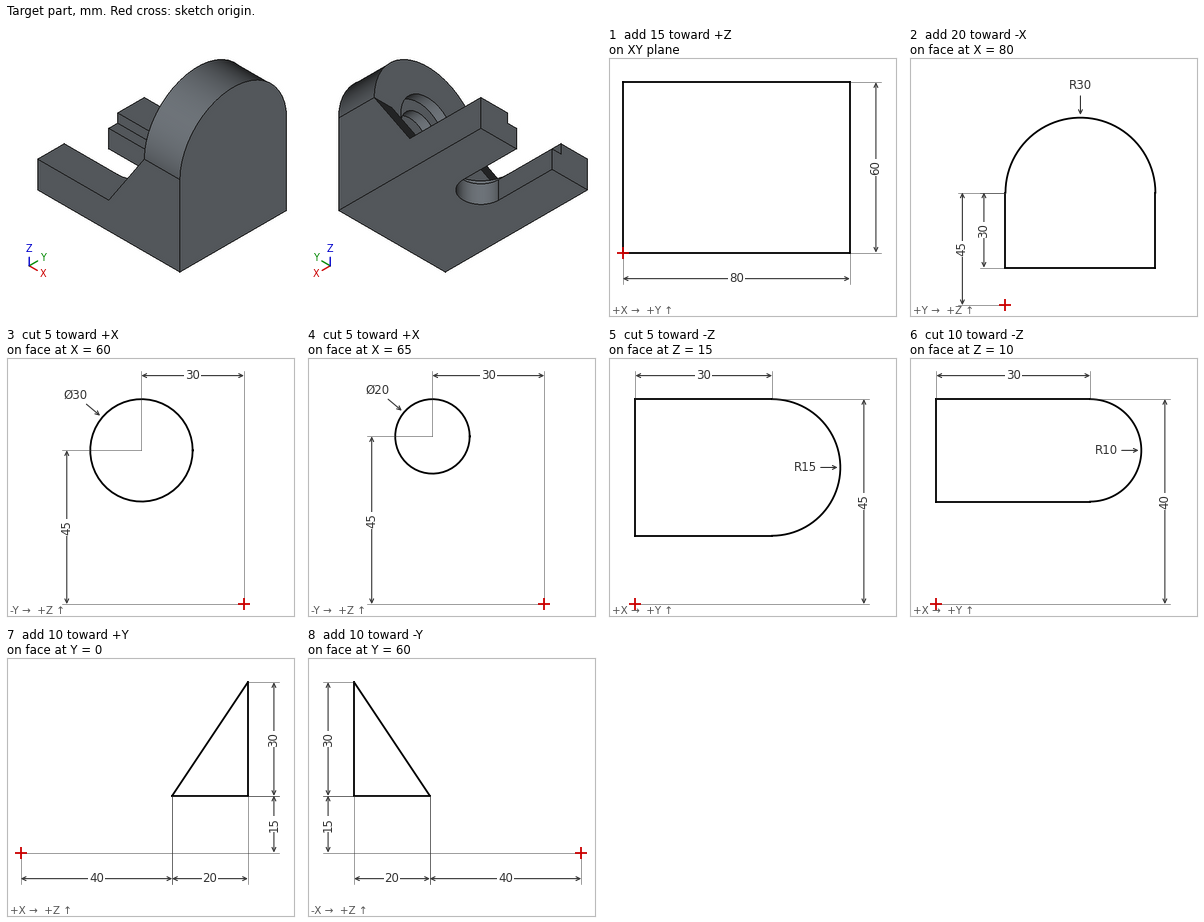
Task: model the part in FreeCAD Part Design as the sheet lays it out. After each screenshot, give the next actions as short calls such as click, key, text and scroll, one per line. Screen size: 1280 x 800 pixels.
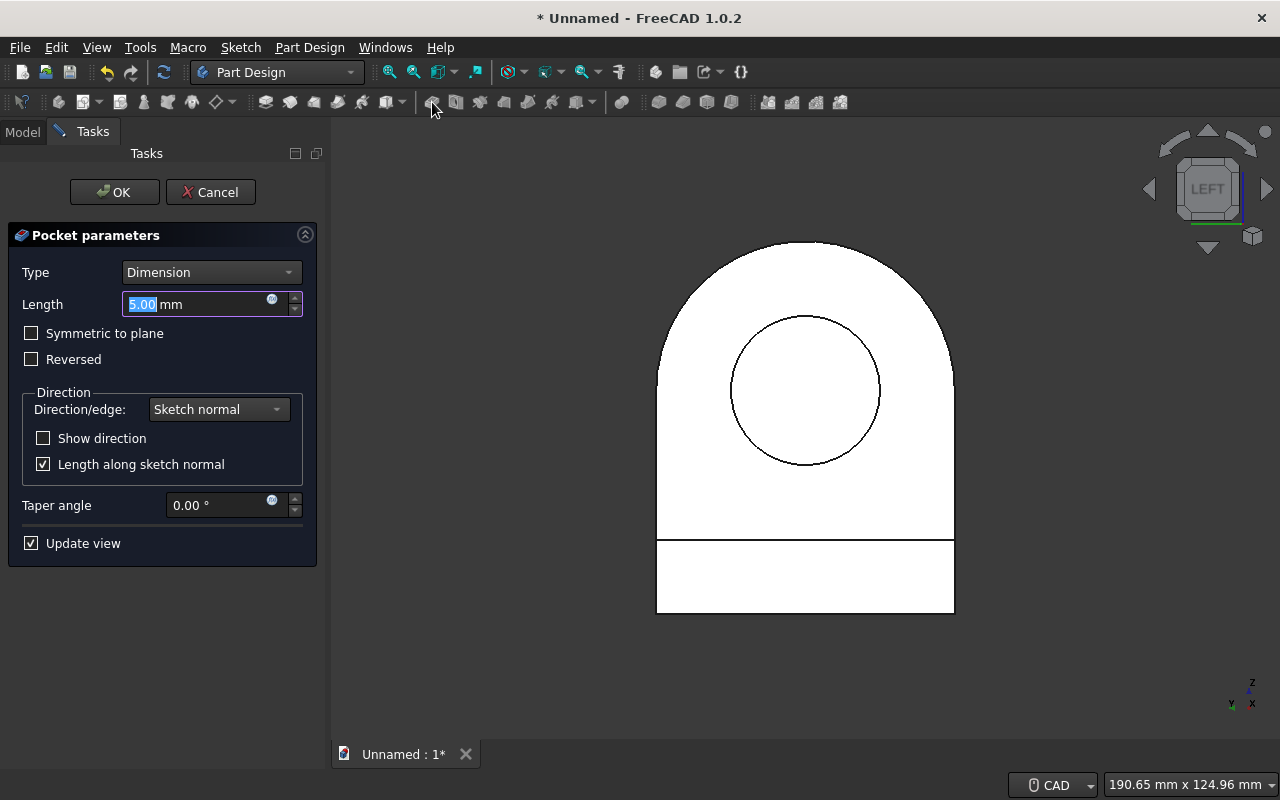
text(5)
key(Tab)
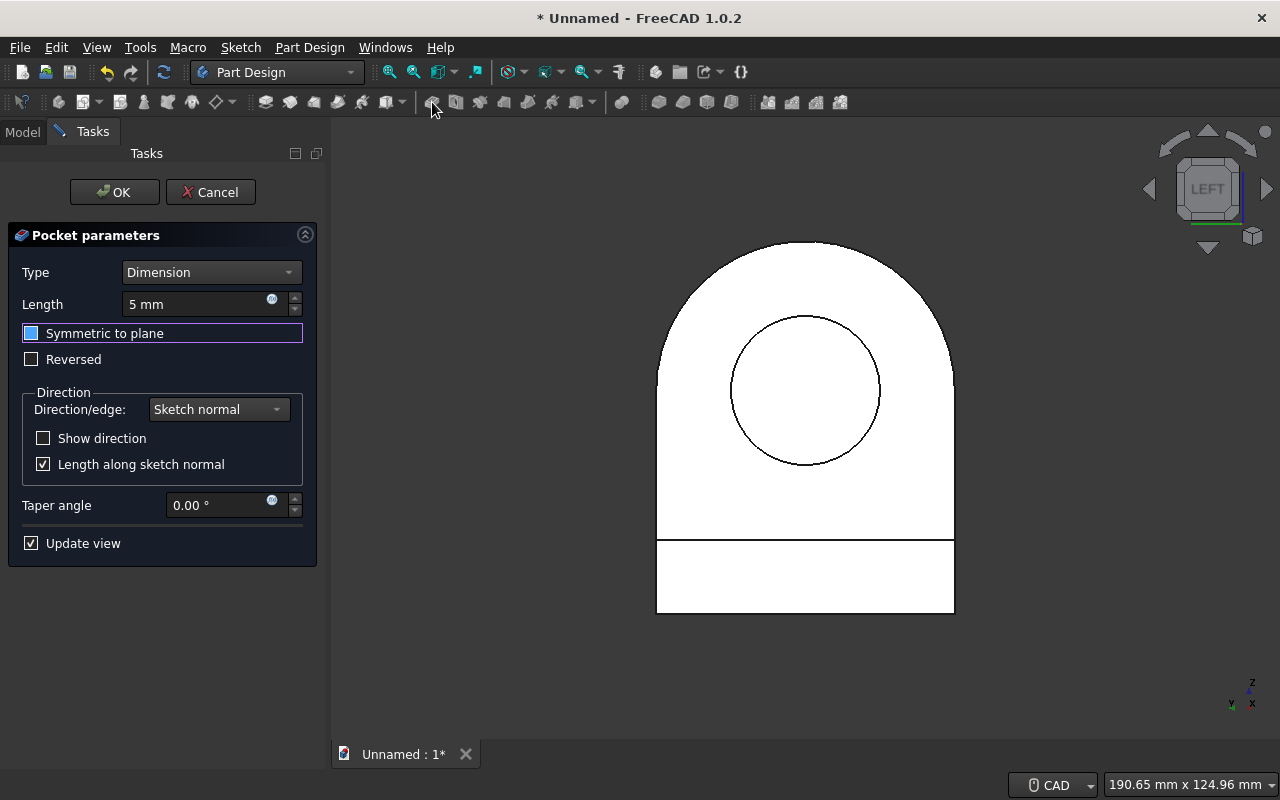
click(115, 192)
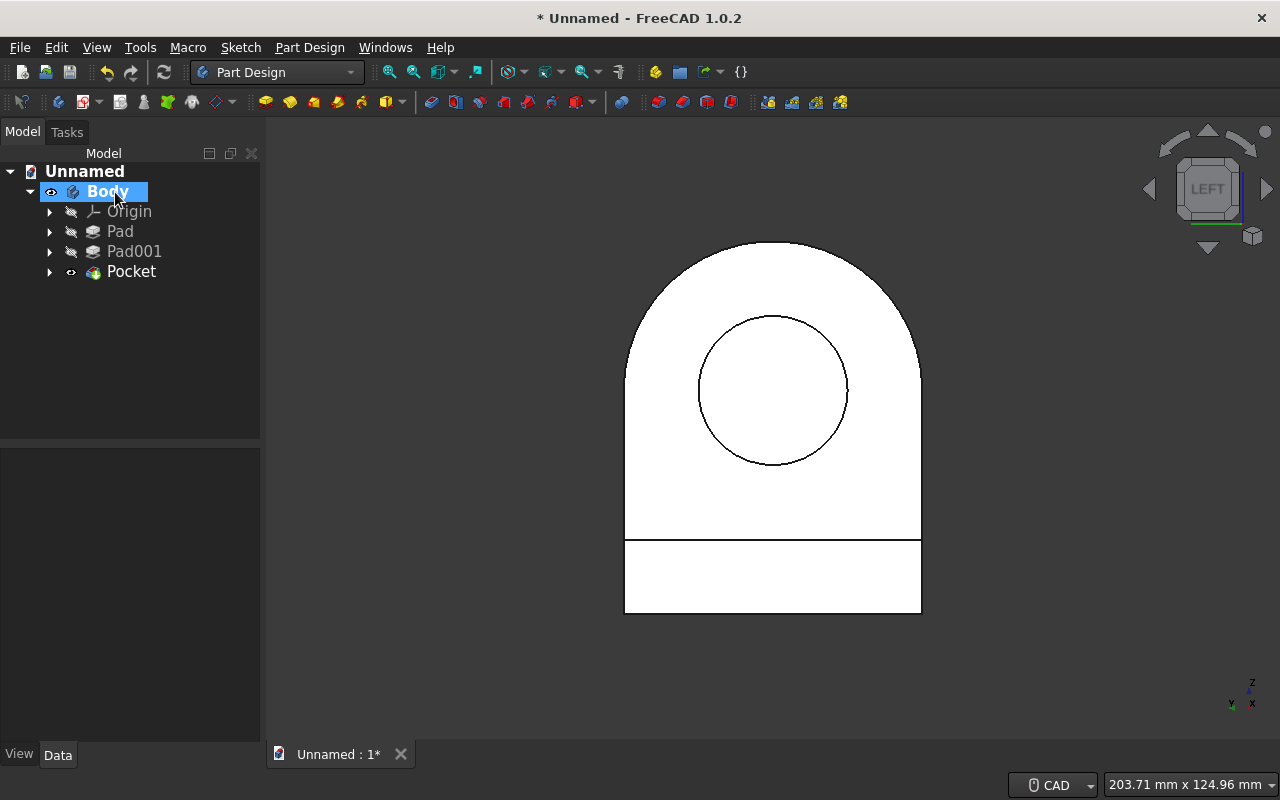
click(773, 389)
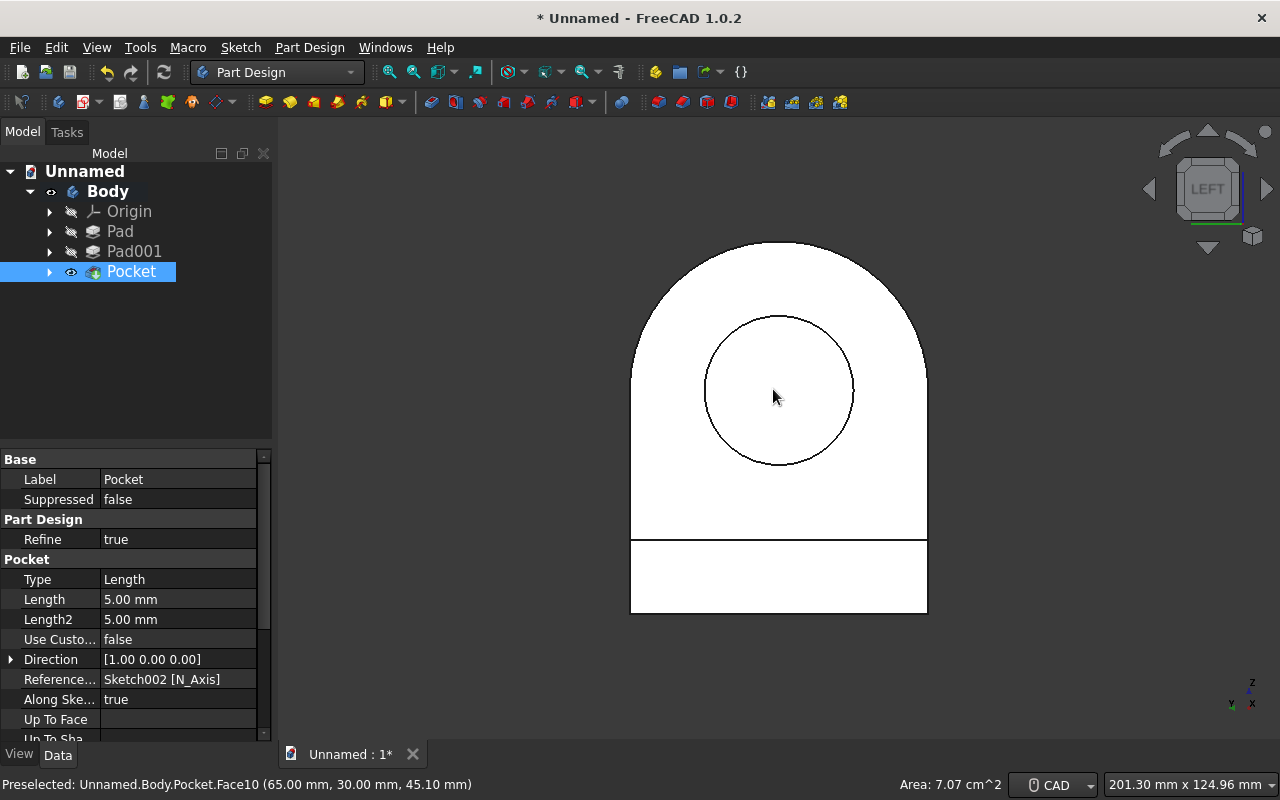
click(84, 102)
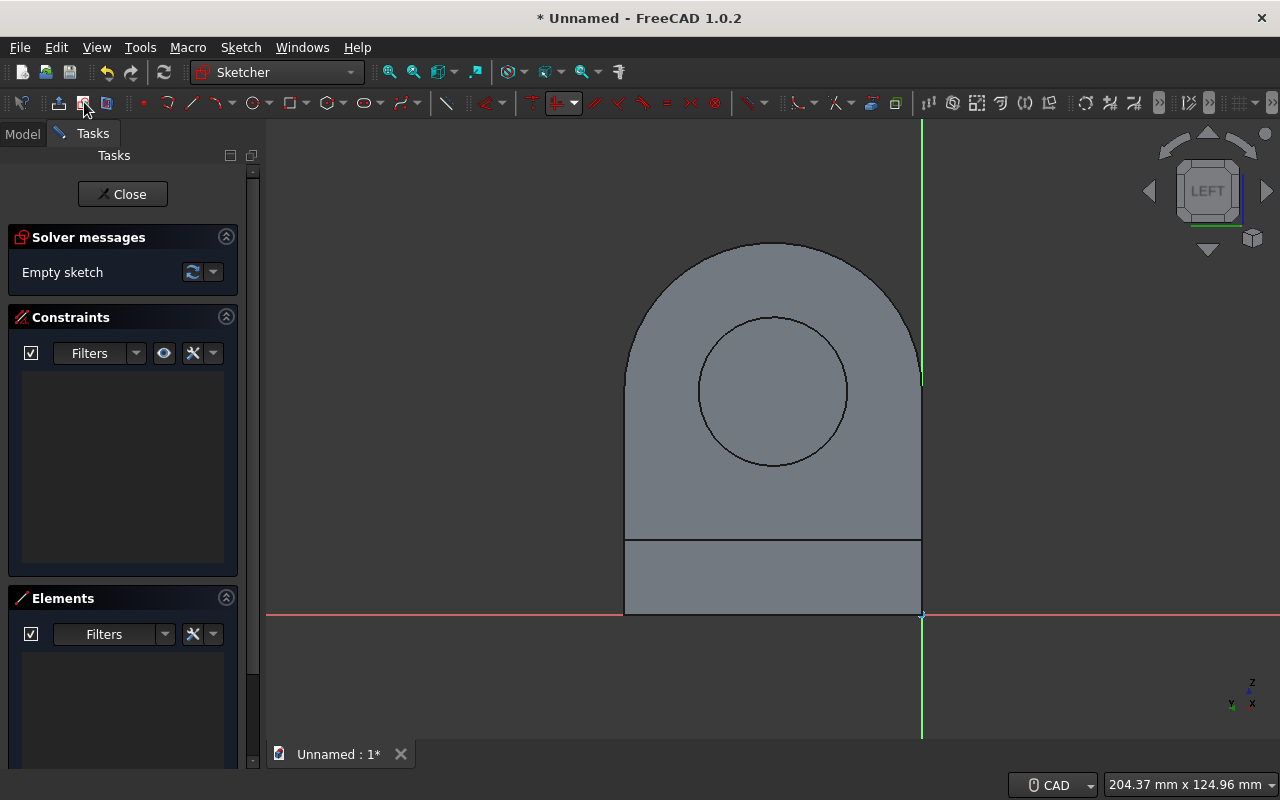
scroll(795, 379, up, 7)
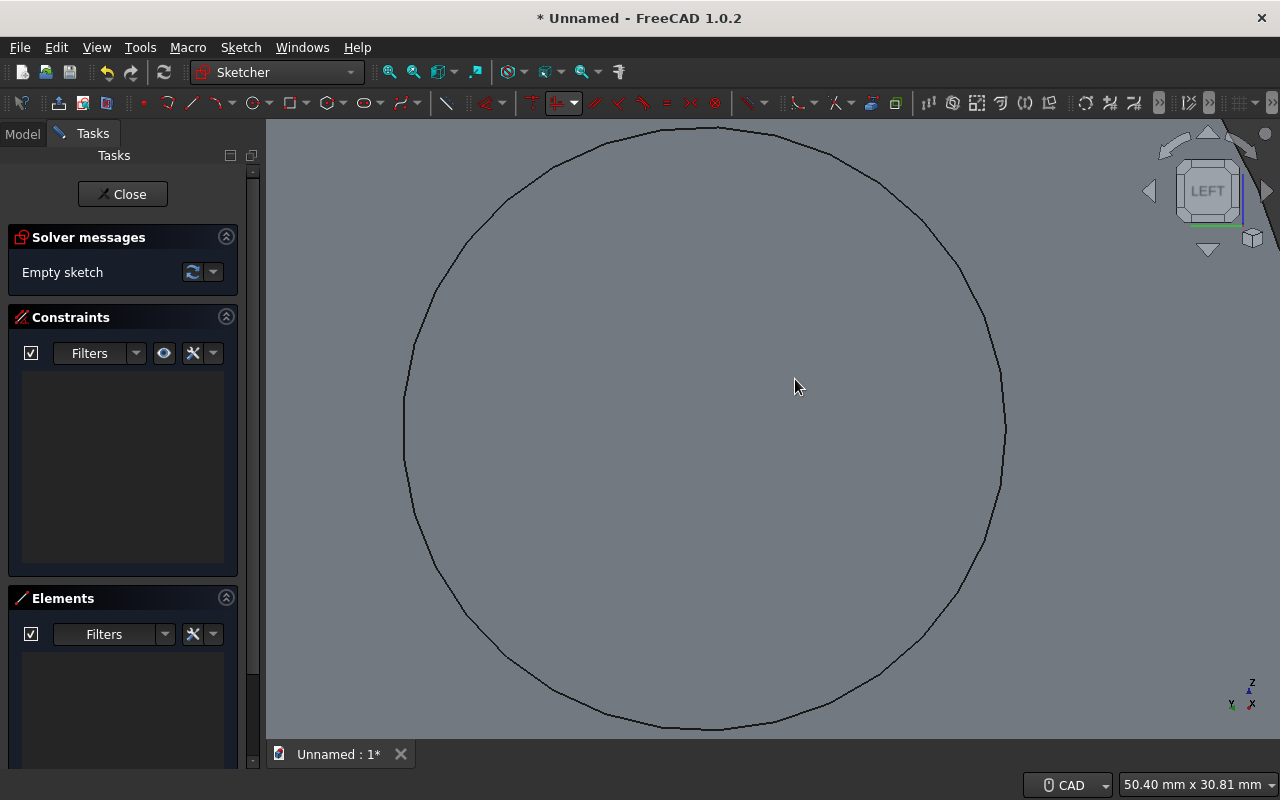
click(254, 104)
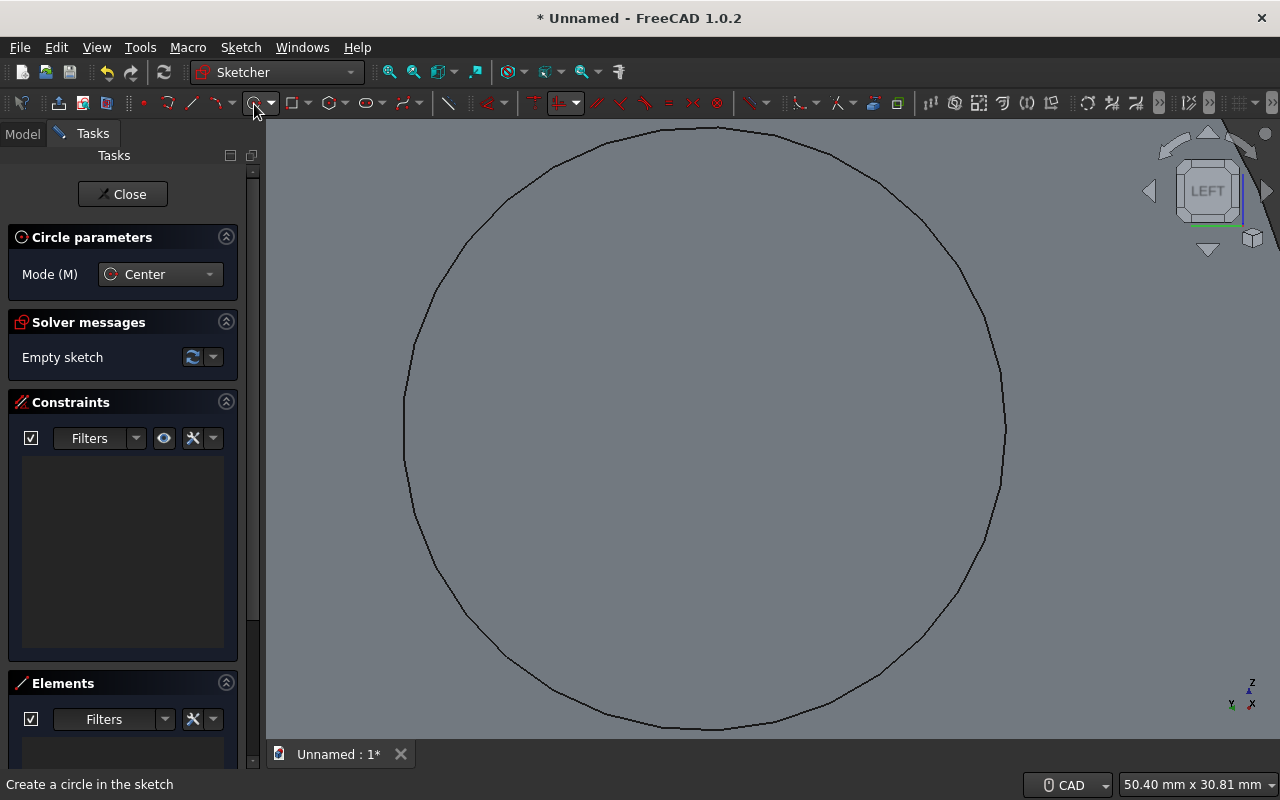
click(704, 429)
click(846, 287)
key(Escape)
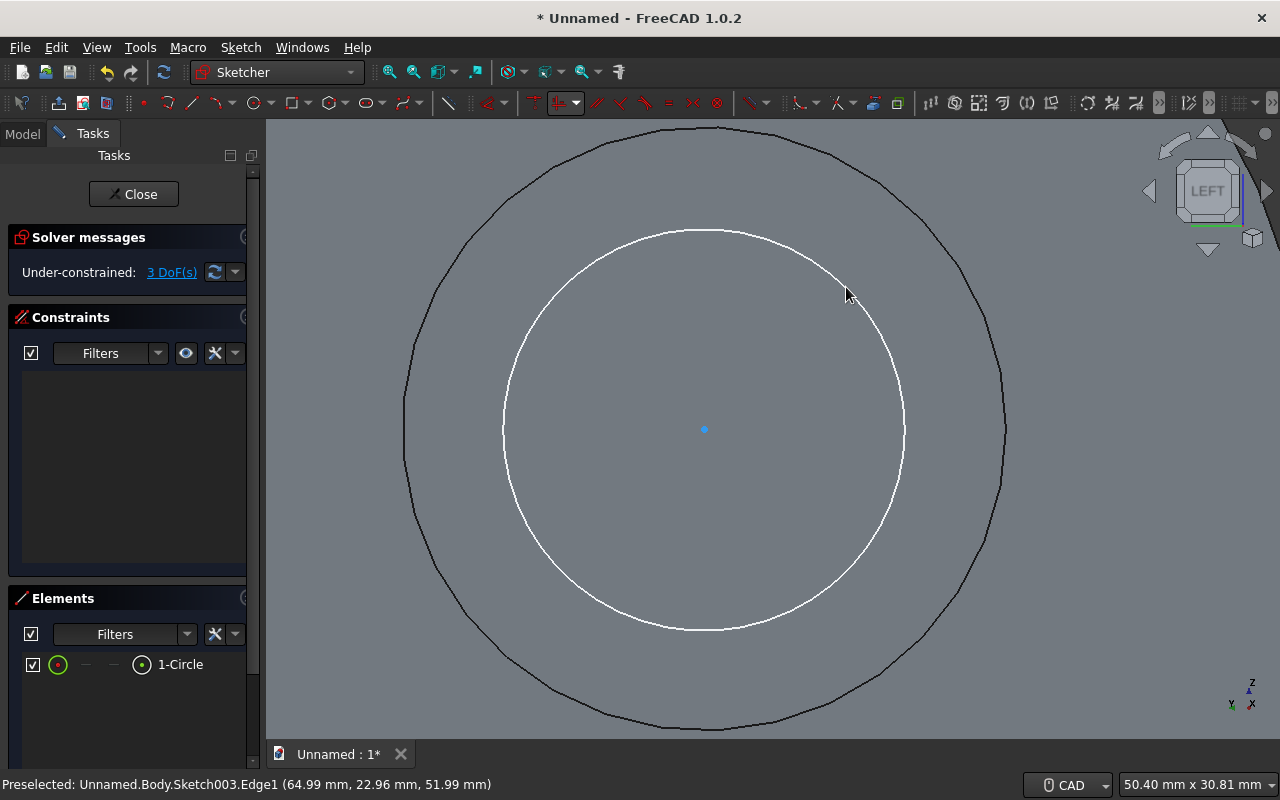
click(488, 104)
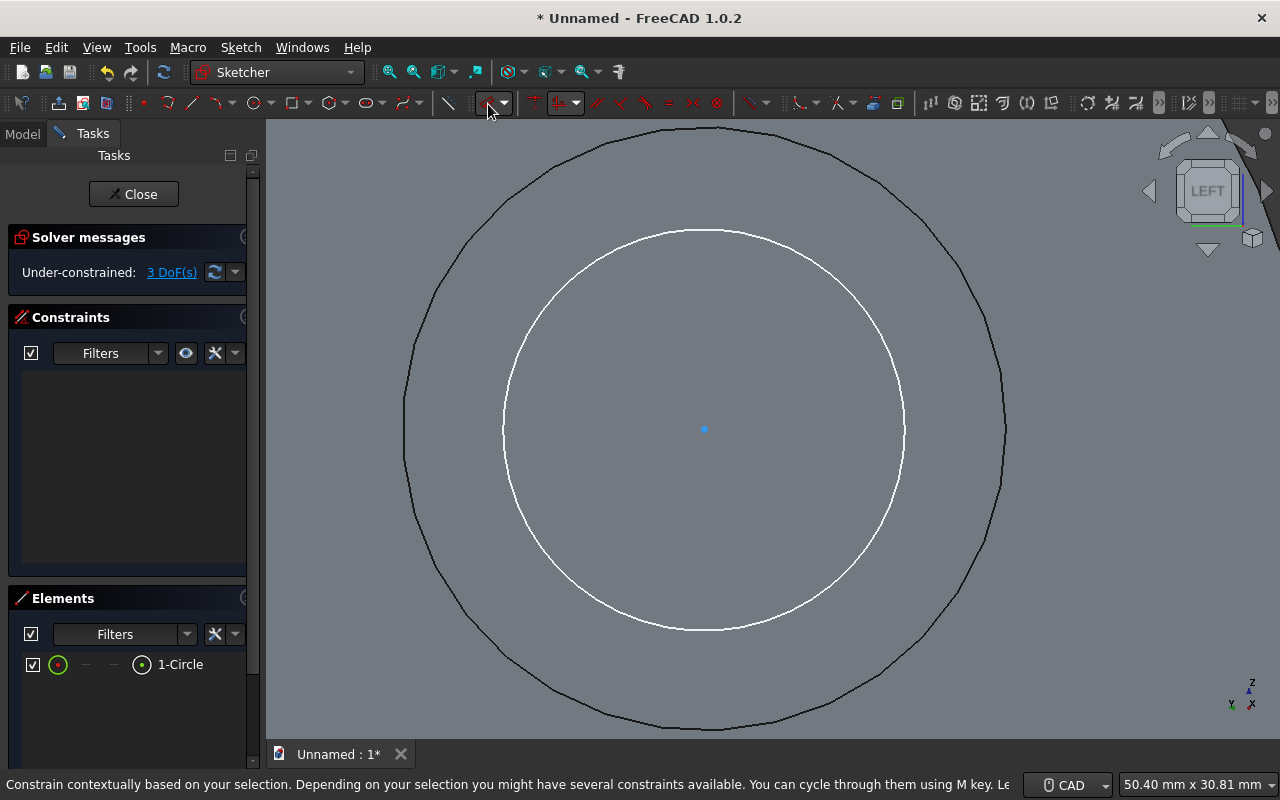
click(846, 288)
click(869, 265)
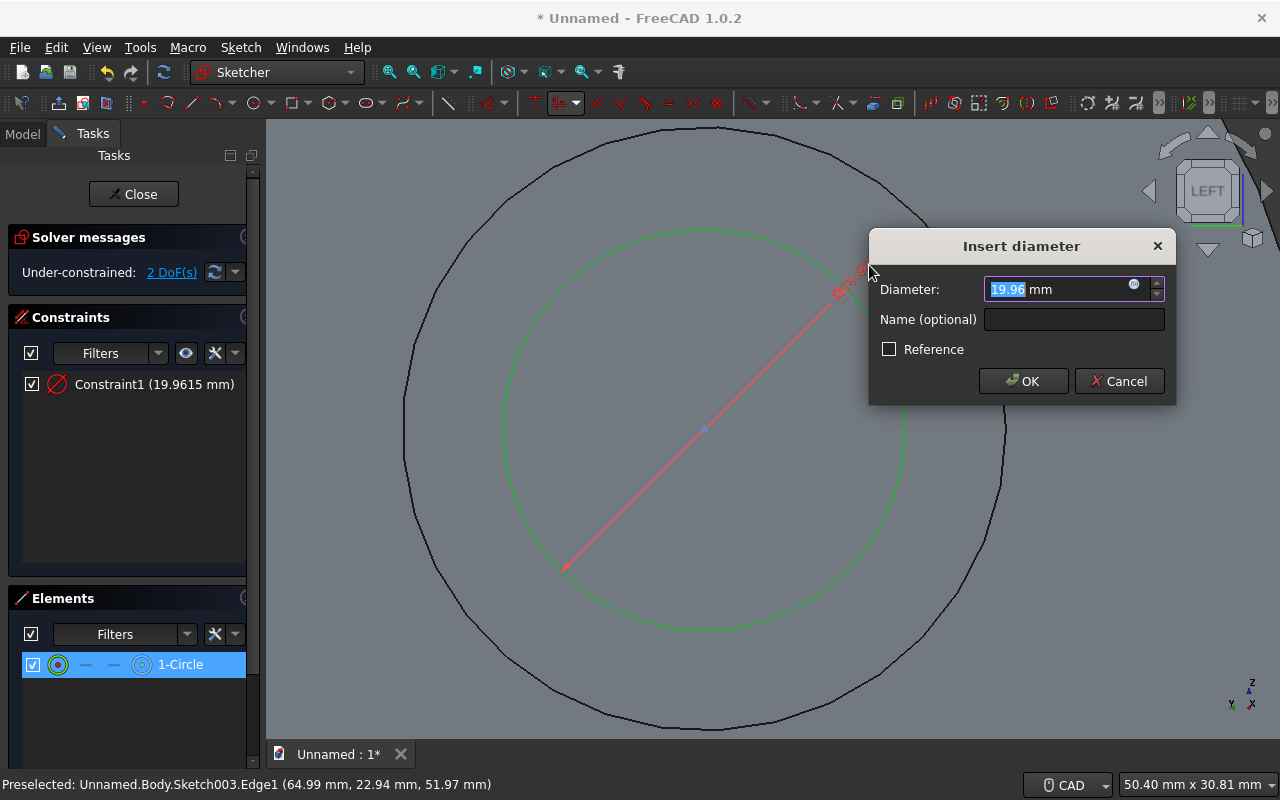
text(20)
key(Return)